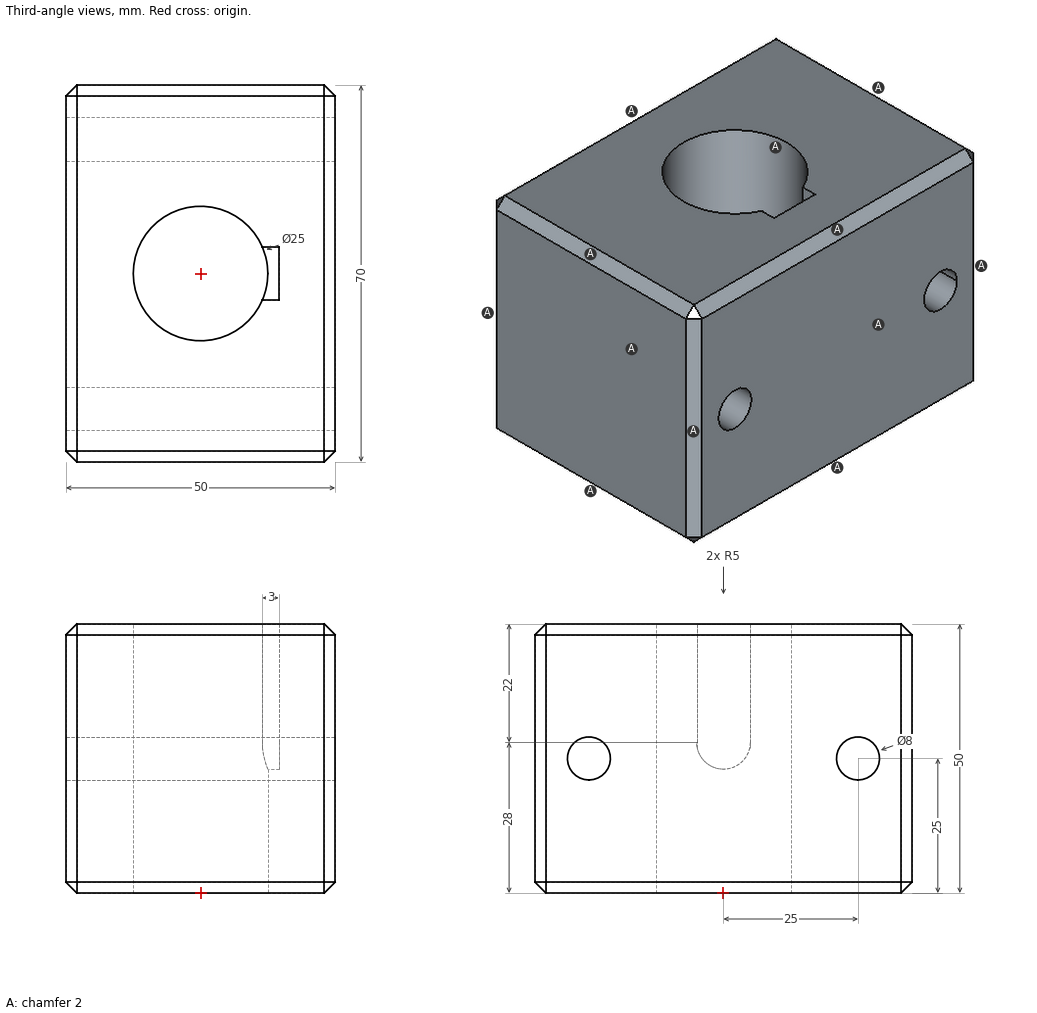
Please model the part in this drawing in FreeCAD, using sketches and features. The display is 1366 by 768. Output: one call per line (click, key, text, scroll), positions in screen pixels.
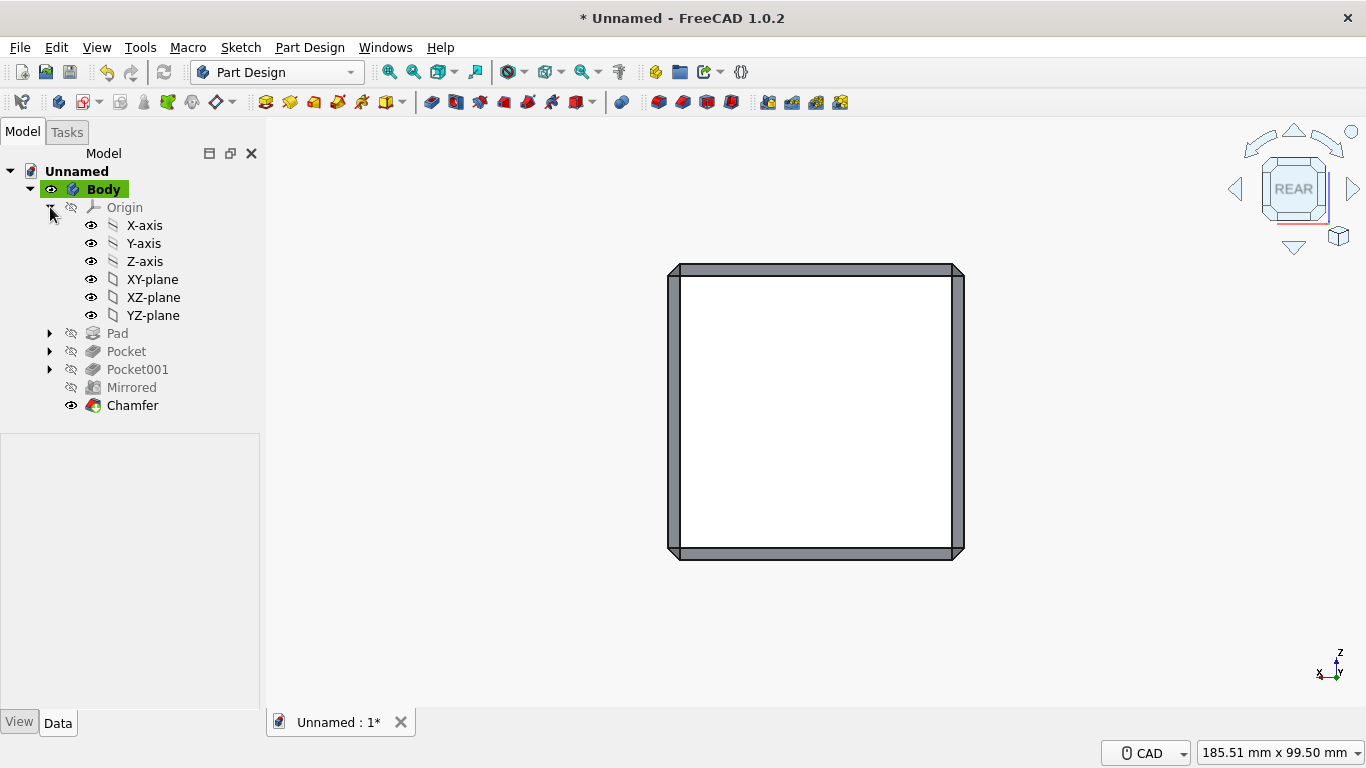
click(136, 315)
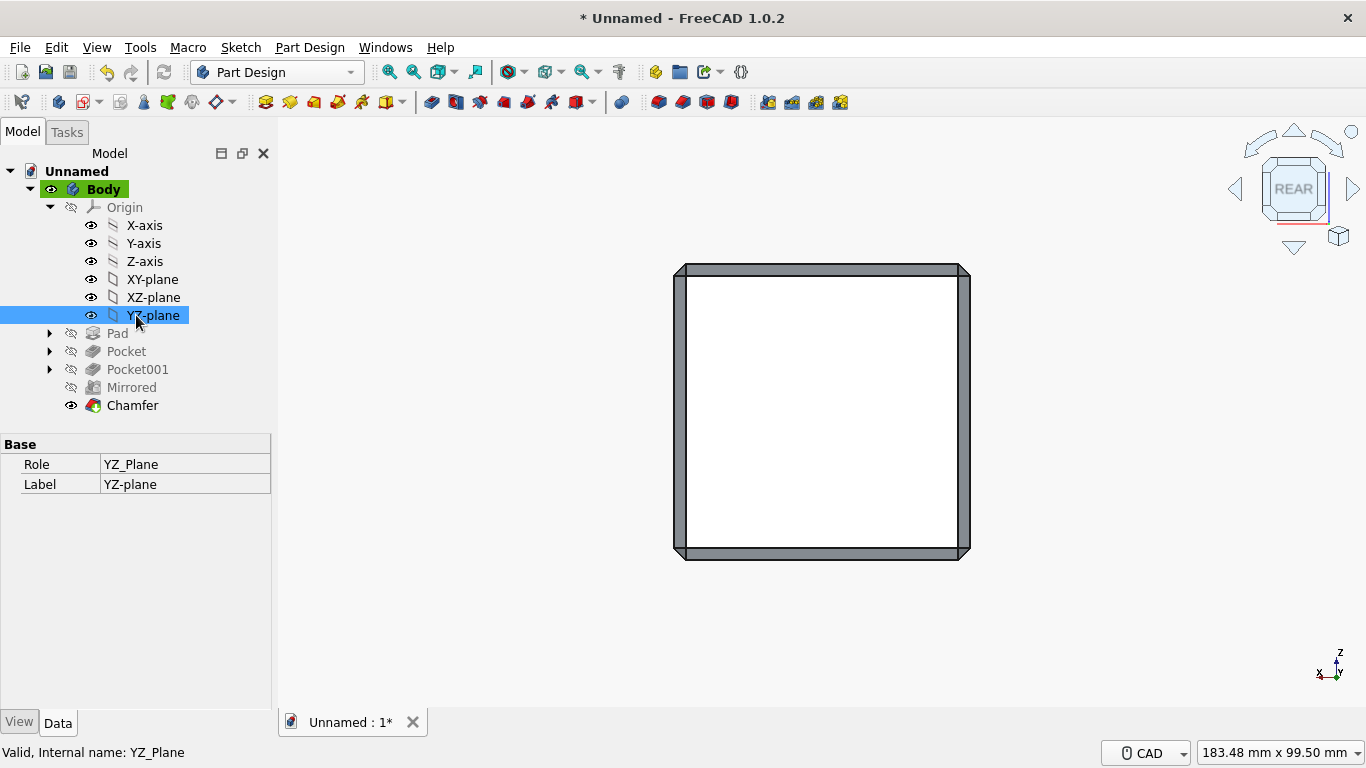
click(216, 102)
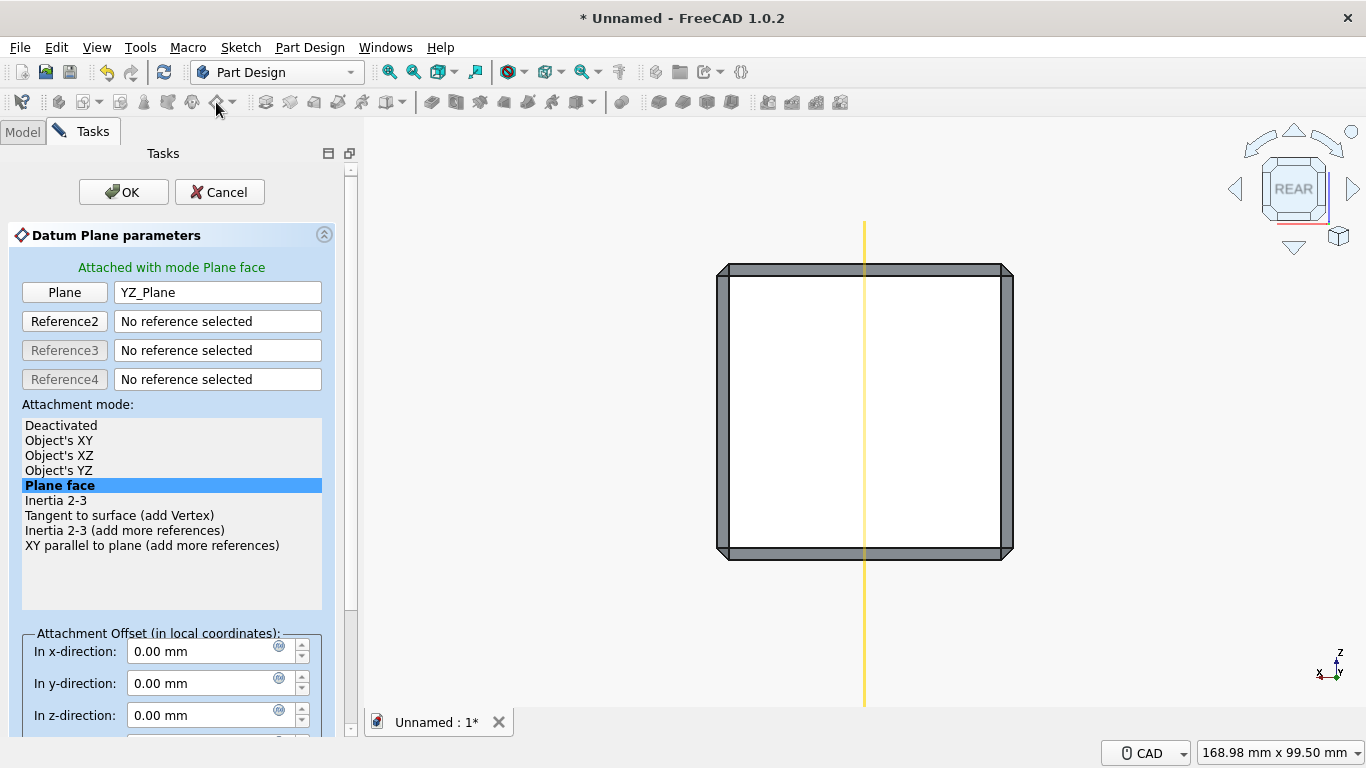
triple_click(210, 715)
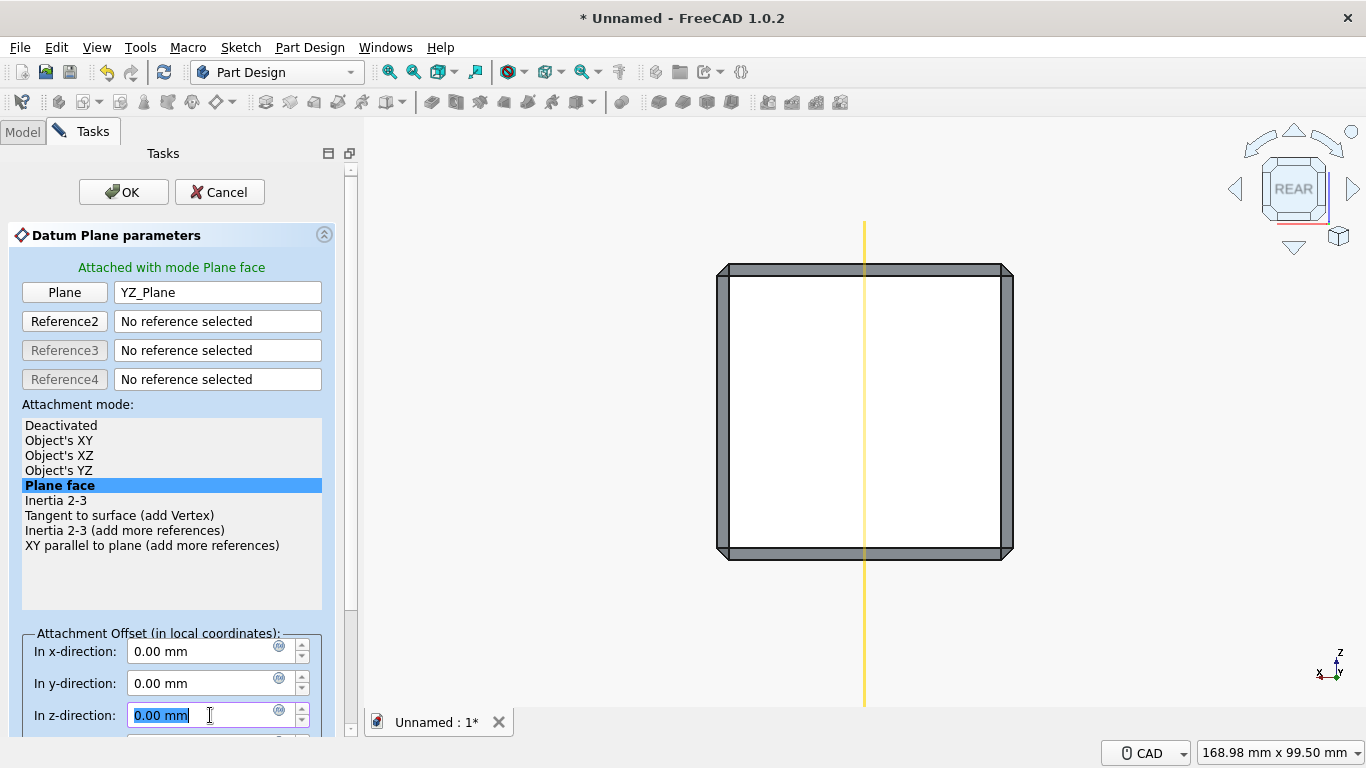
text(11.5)
key(Tab)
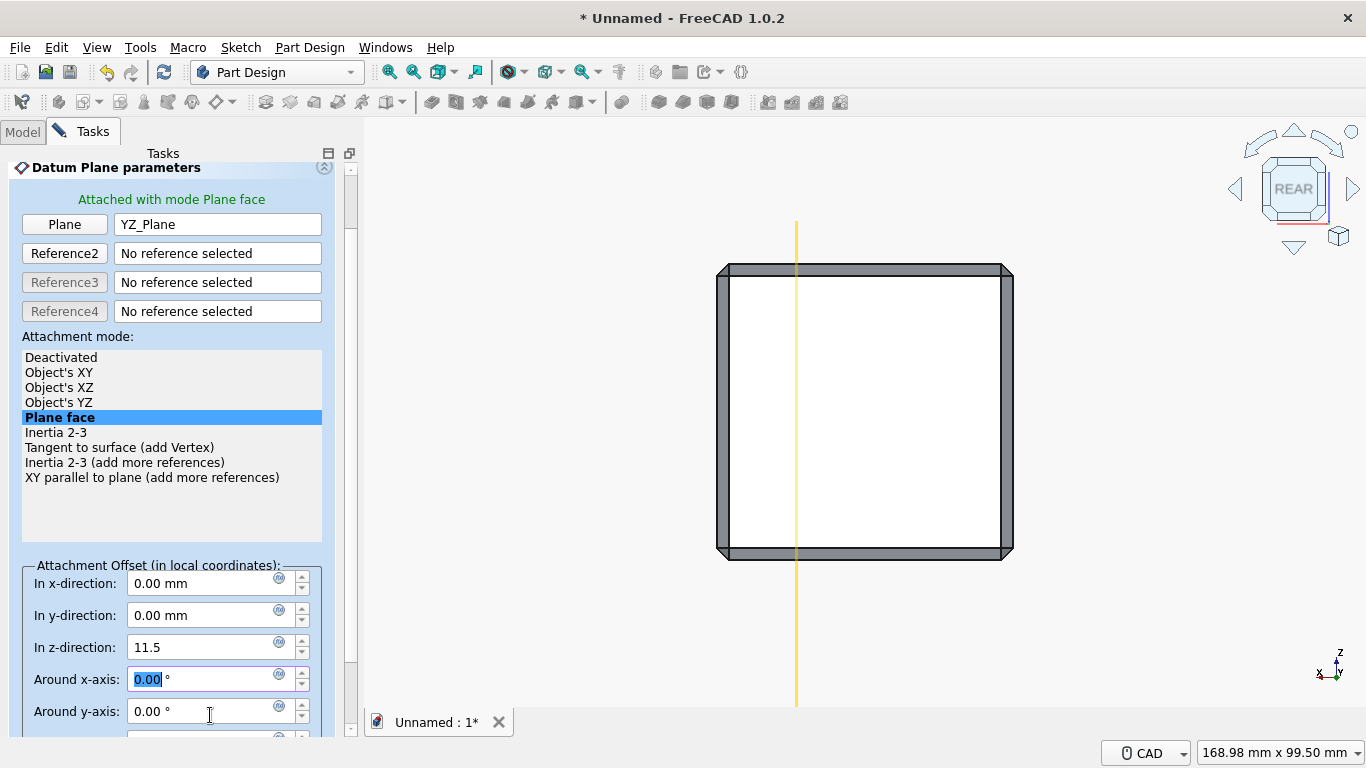
scroll(351, 450, up, 2)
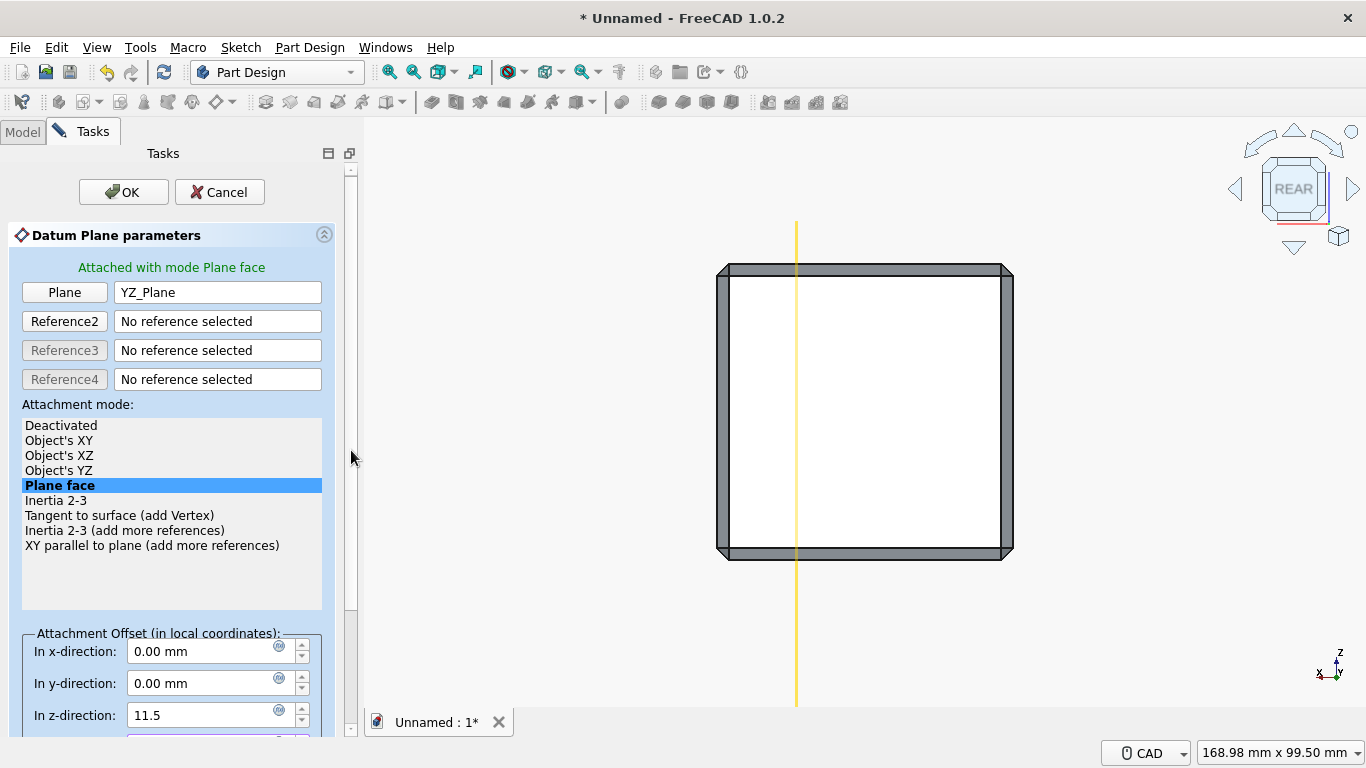
click(124, 192)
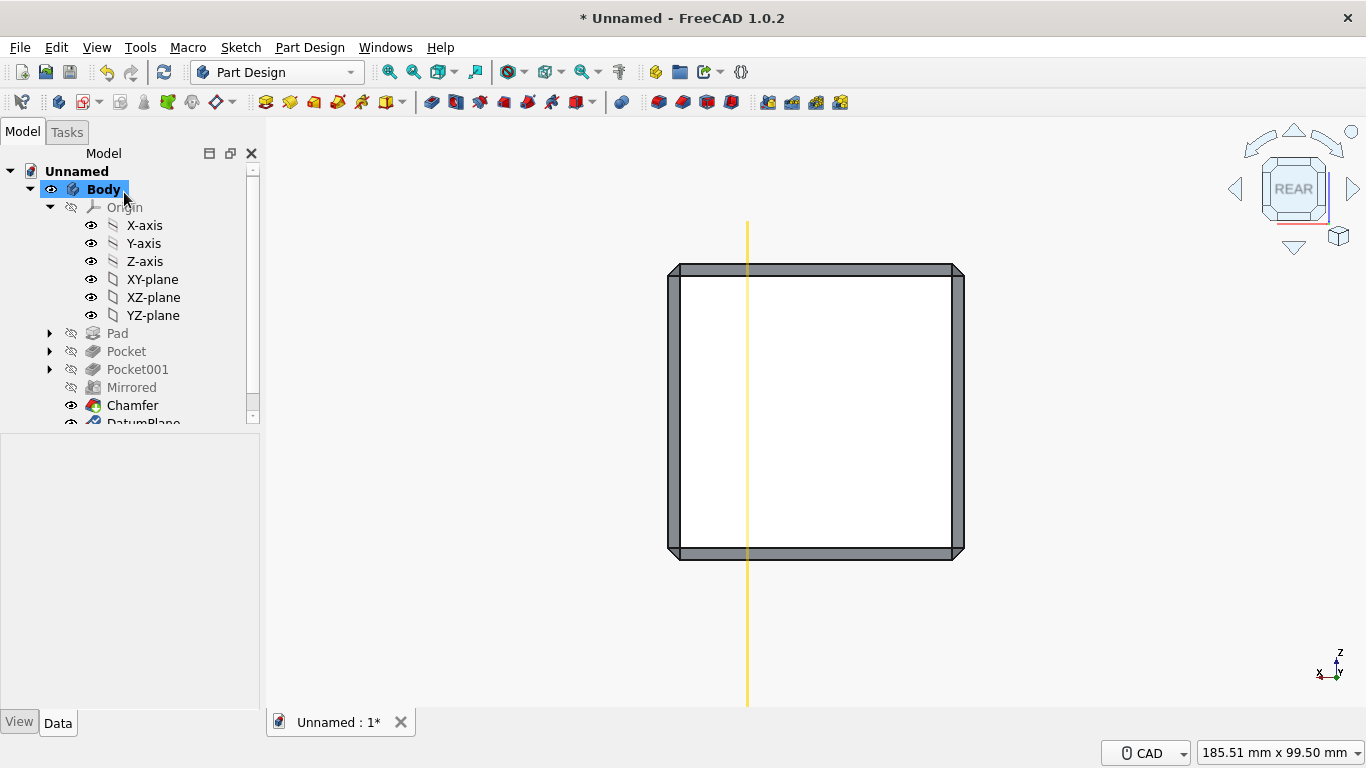
click(116, 423)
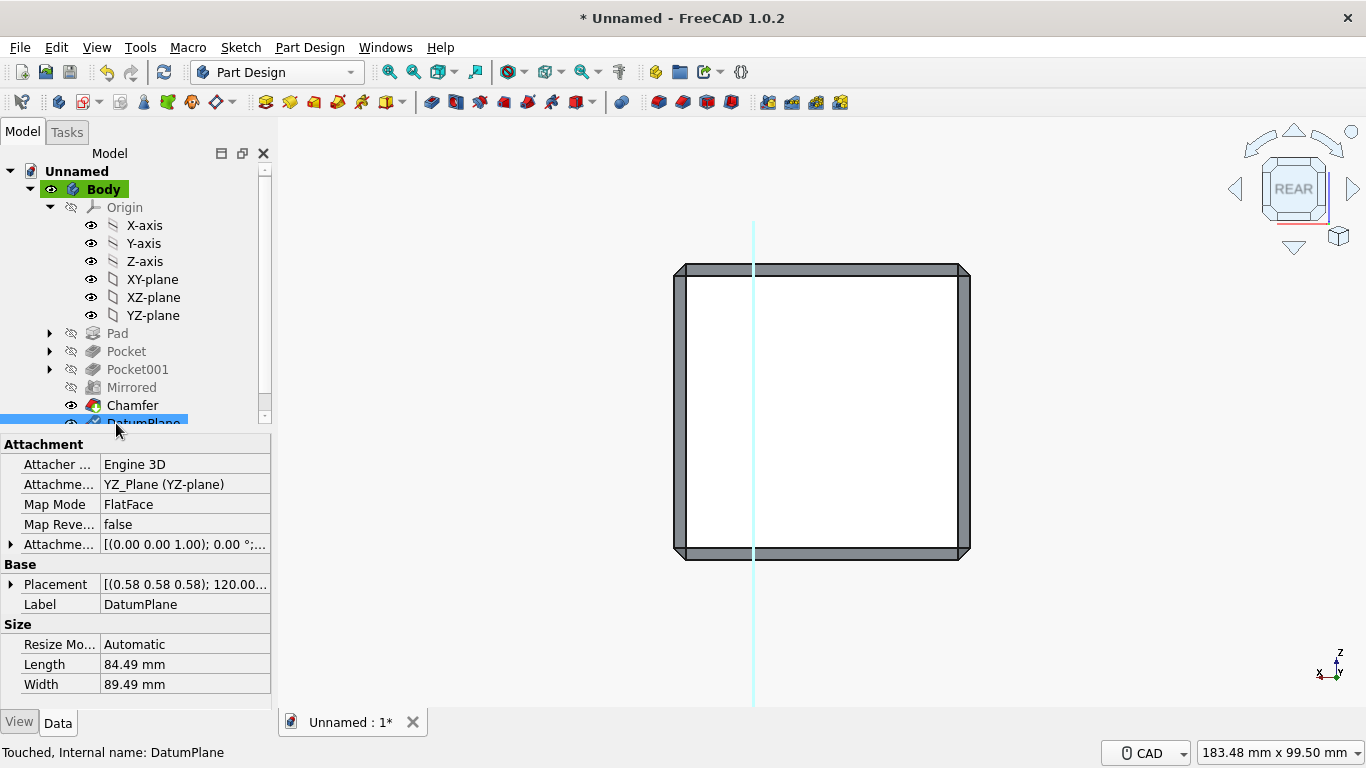
click(84, 102)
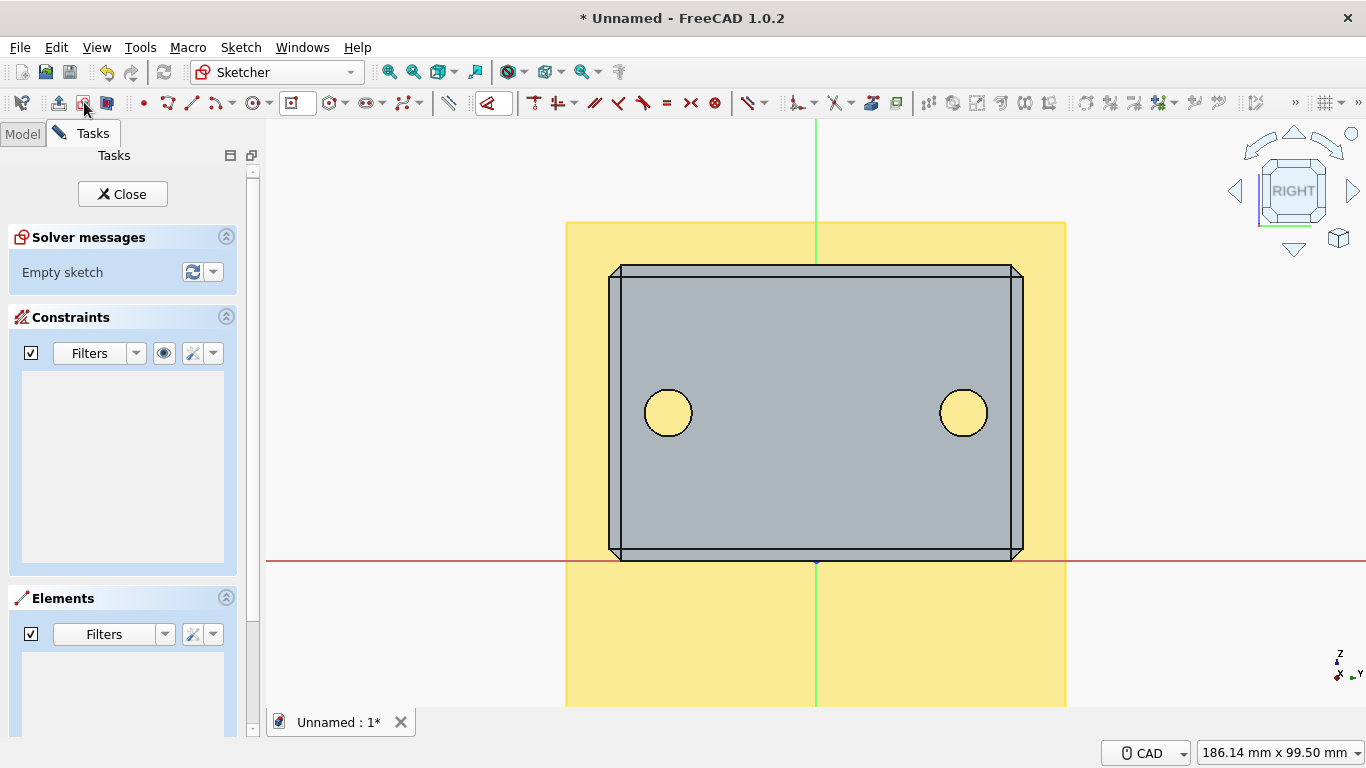
click(108, 104)